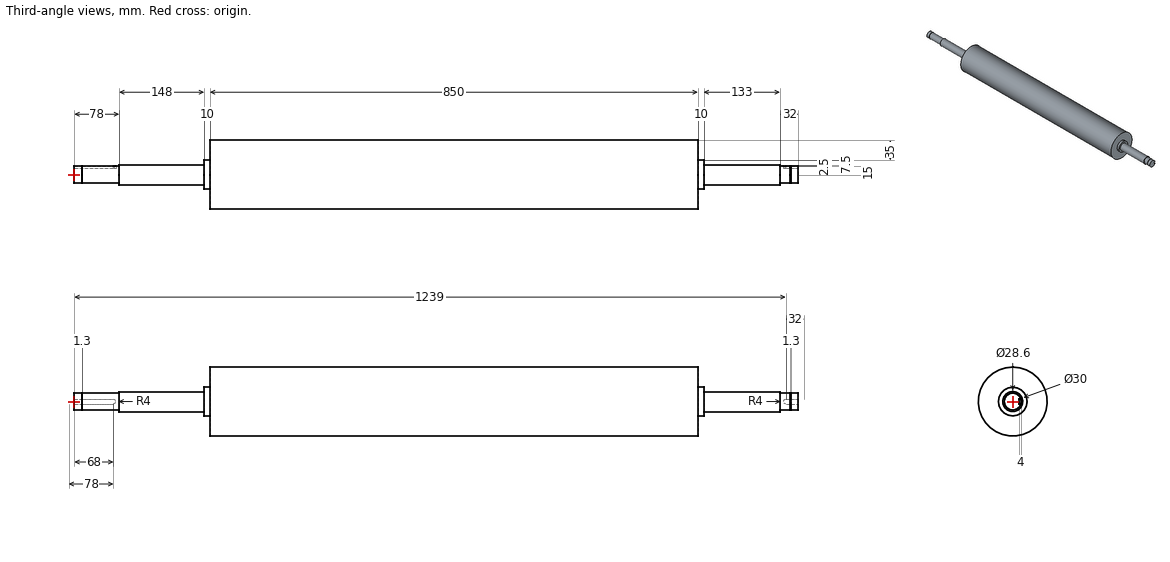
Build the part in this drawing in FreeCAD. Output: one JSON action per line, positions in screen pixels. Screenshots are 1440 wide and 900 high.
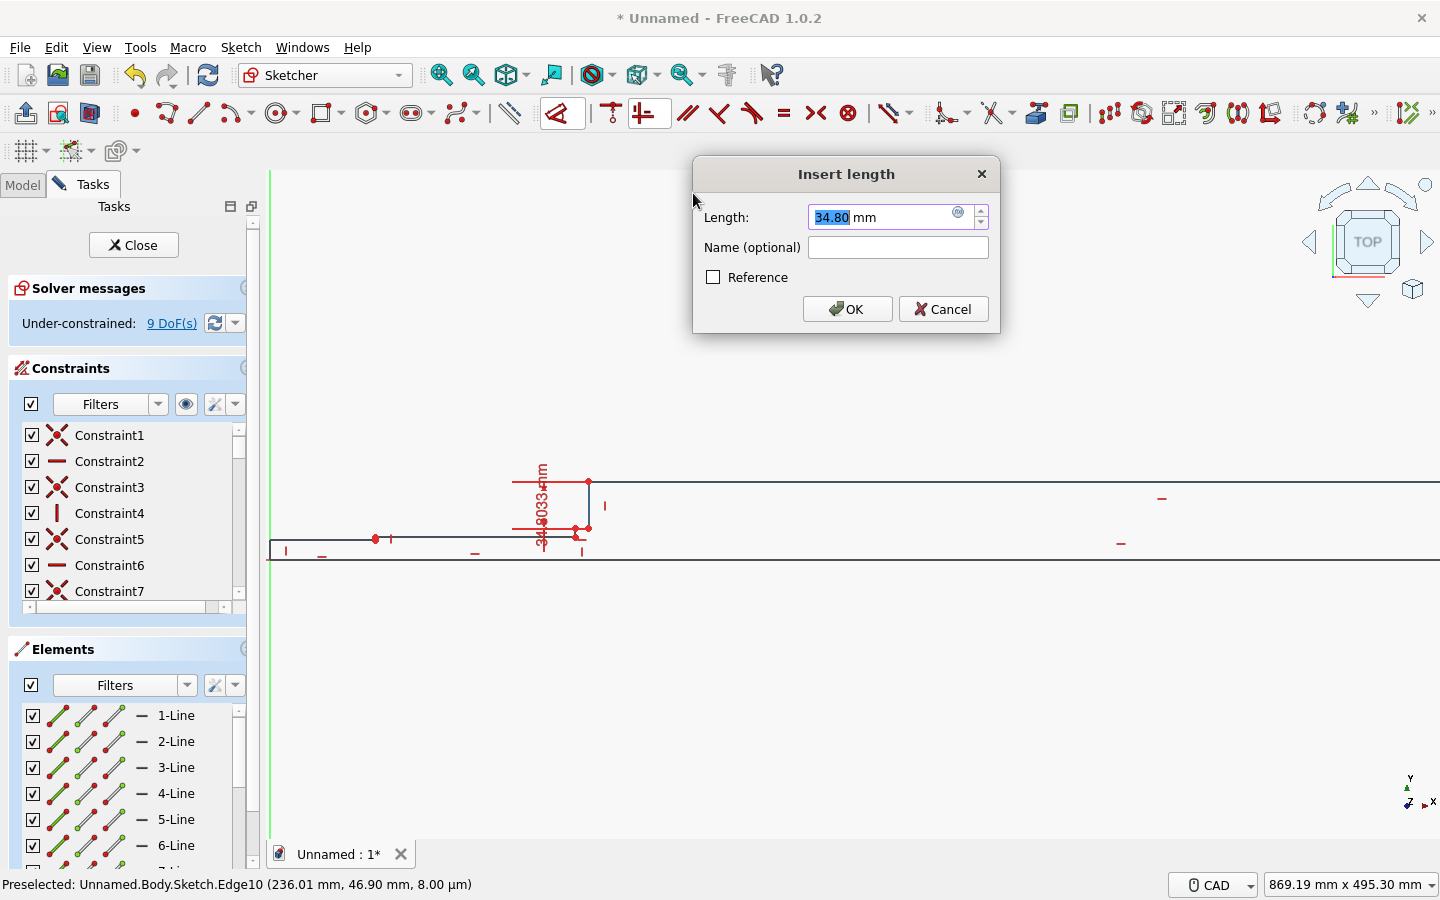
{"action": "type", "text": "35"}
{"action": "key", "text": "Return"}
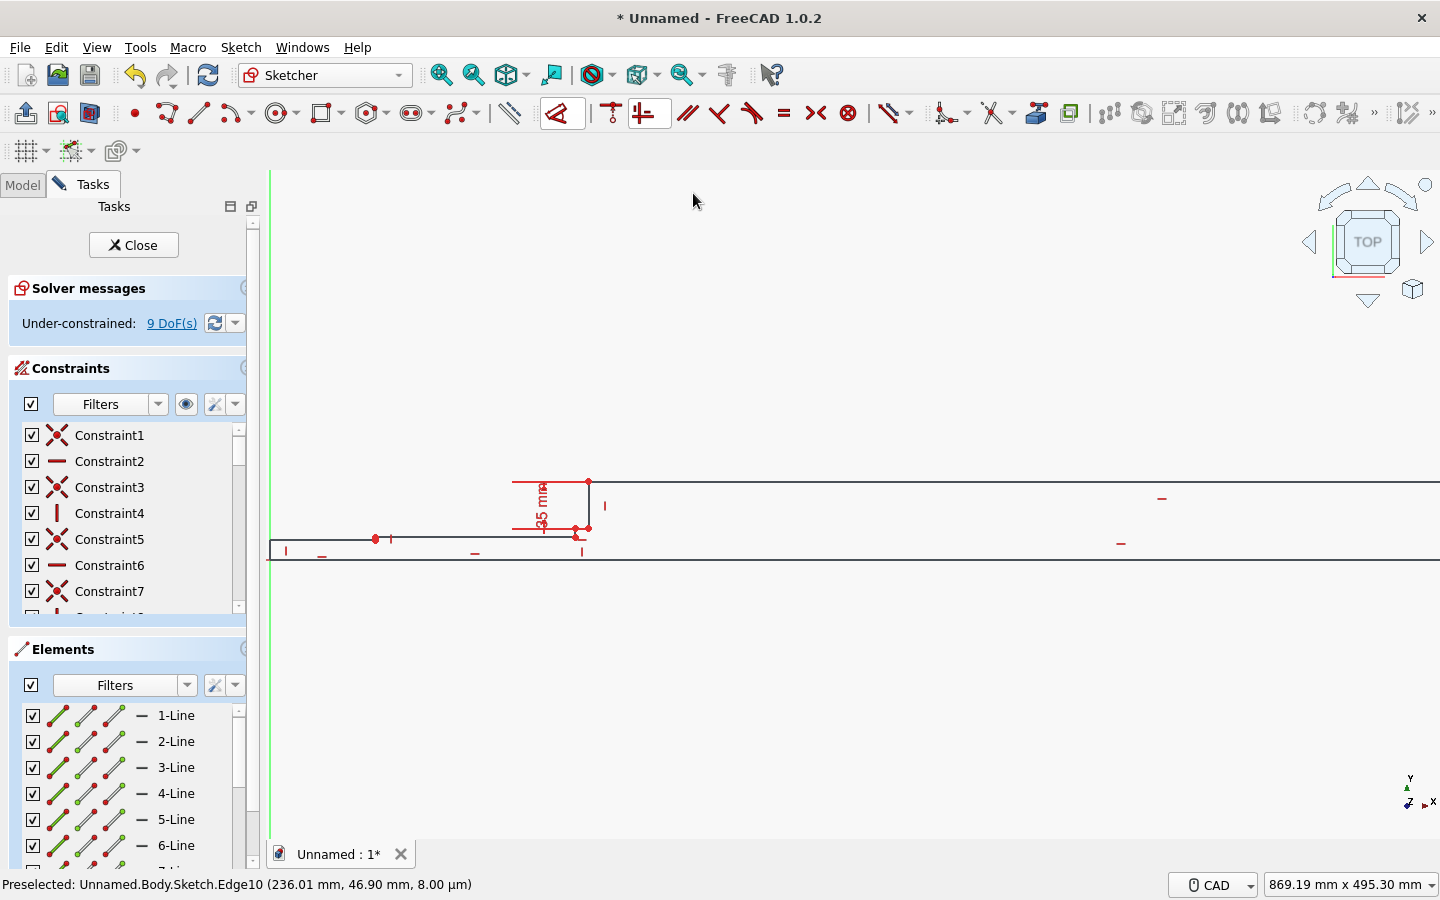
{"action": "scroll", "coordinate": [582, 529], "scroll_direction": "up", "scroll_amount": 6}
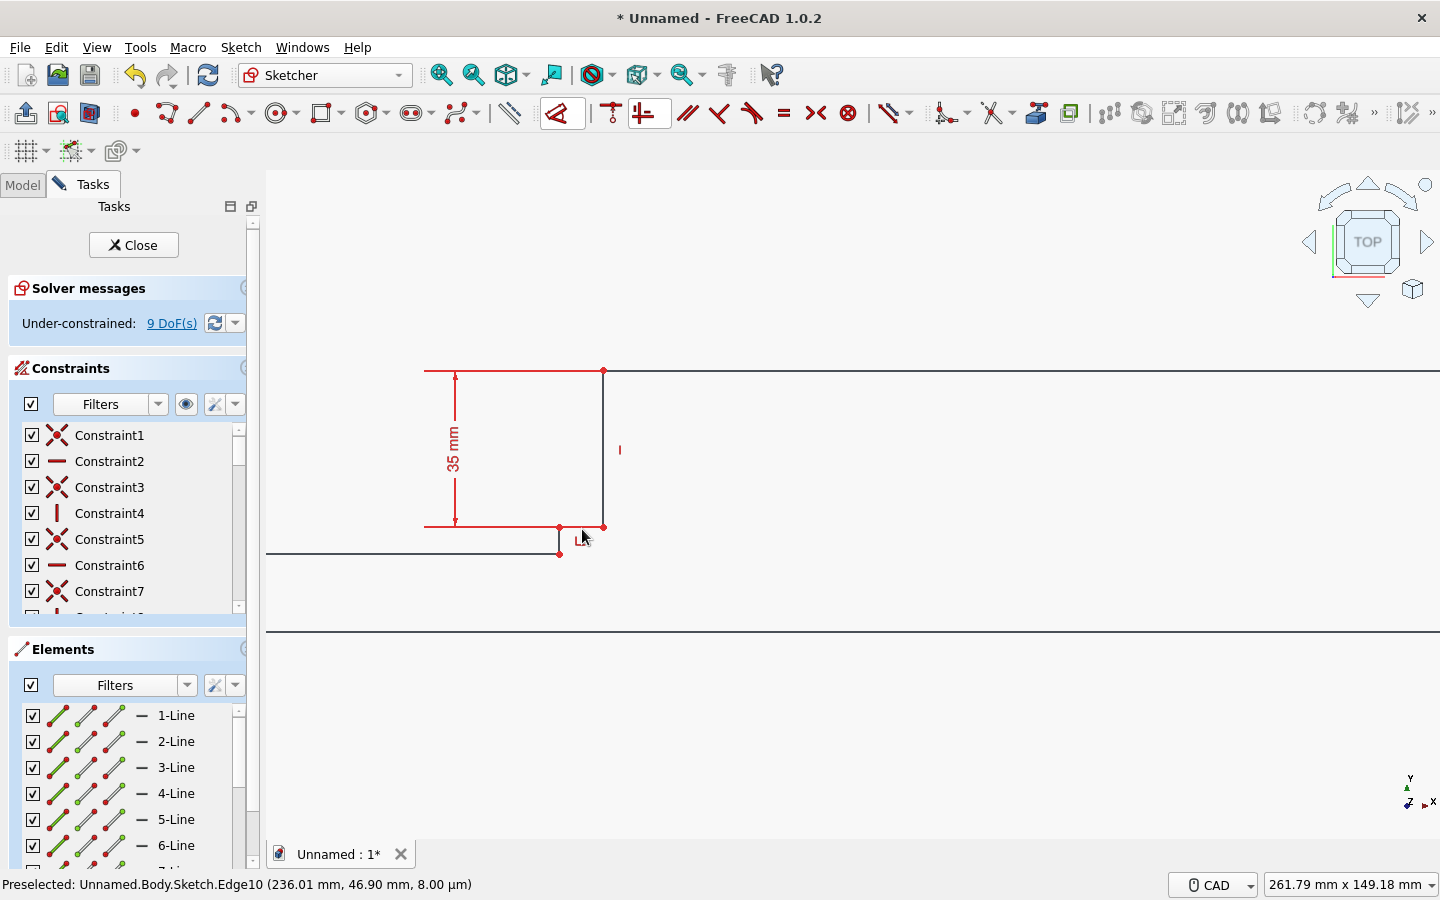
{"action": "left_click", "coordinate": [581, 527]}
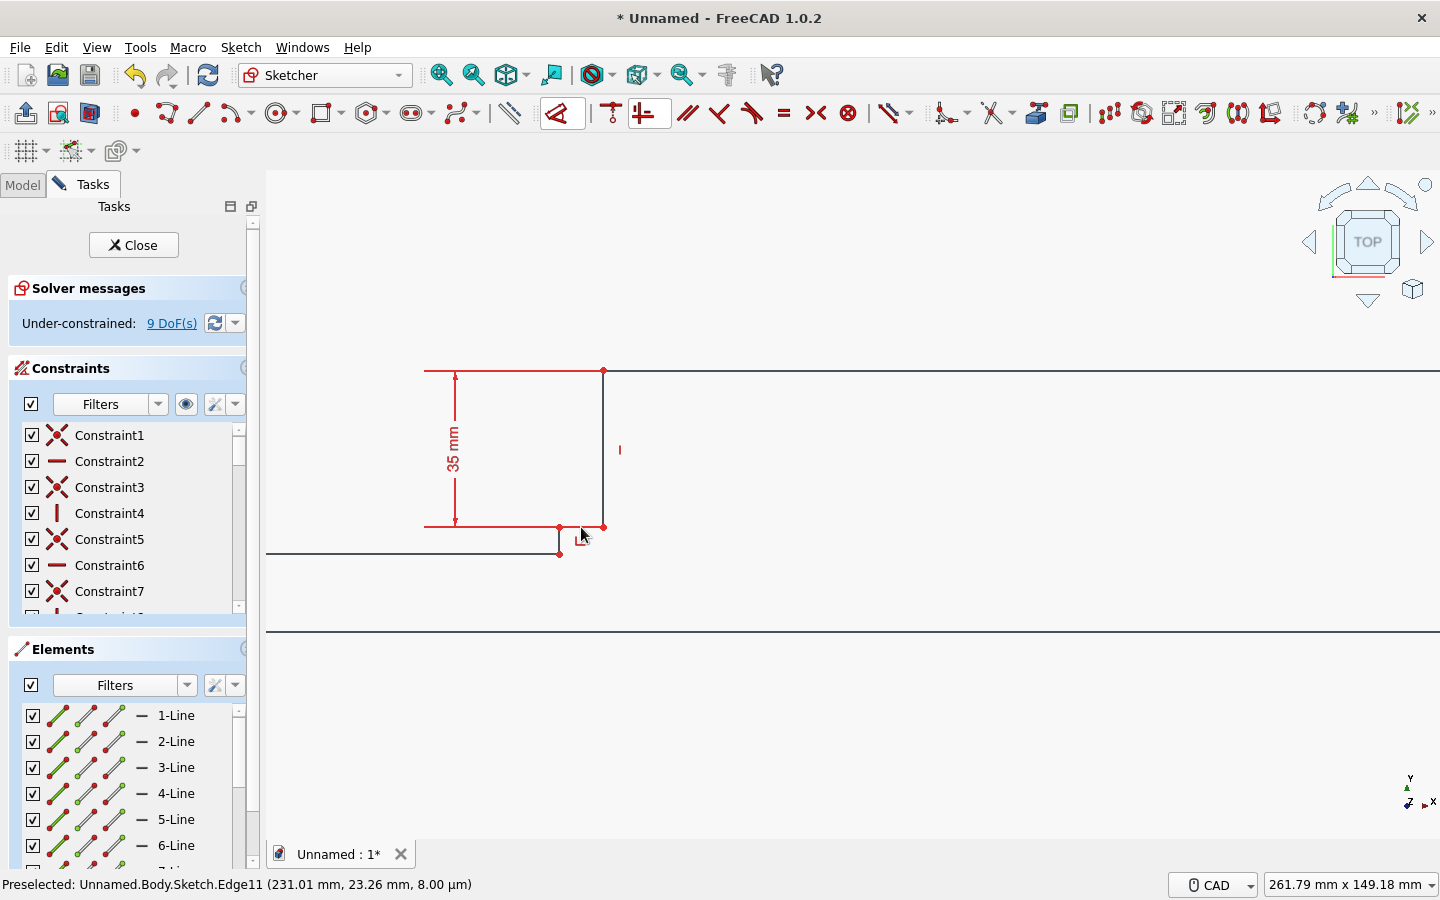
{"action": "key", "text": "l"}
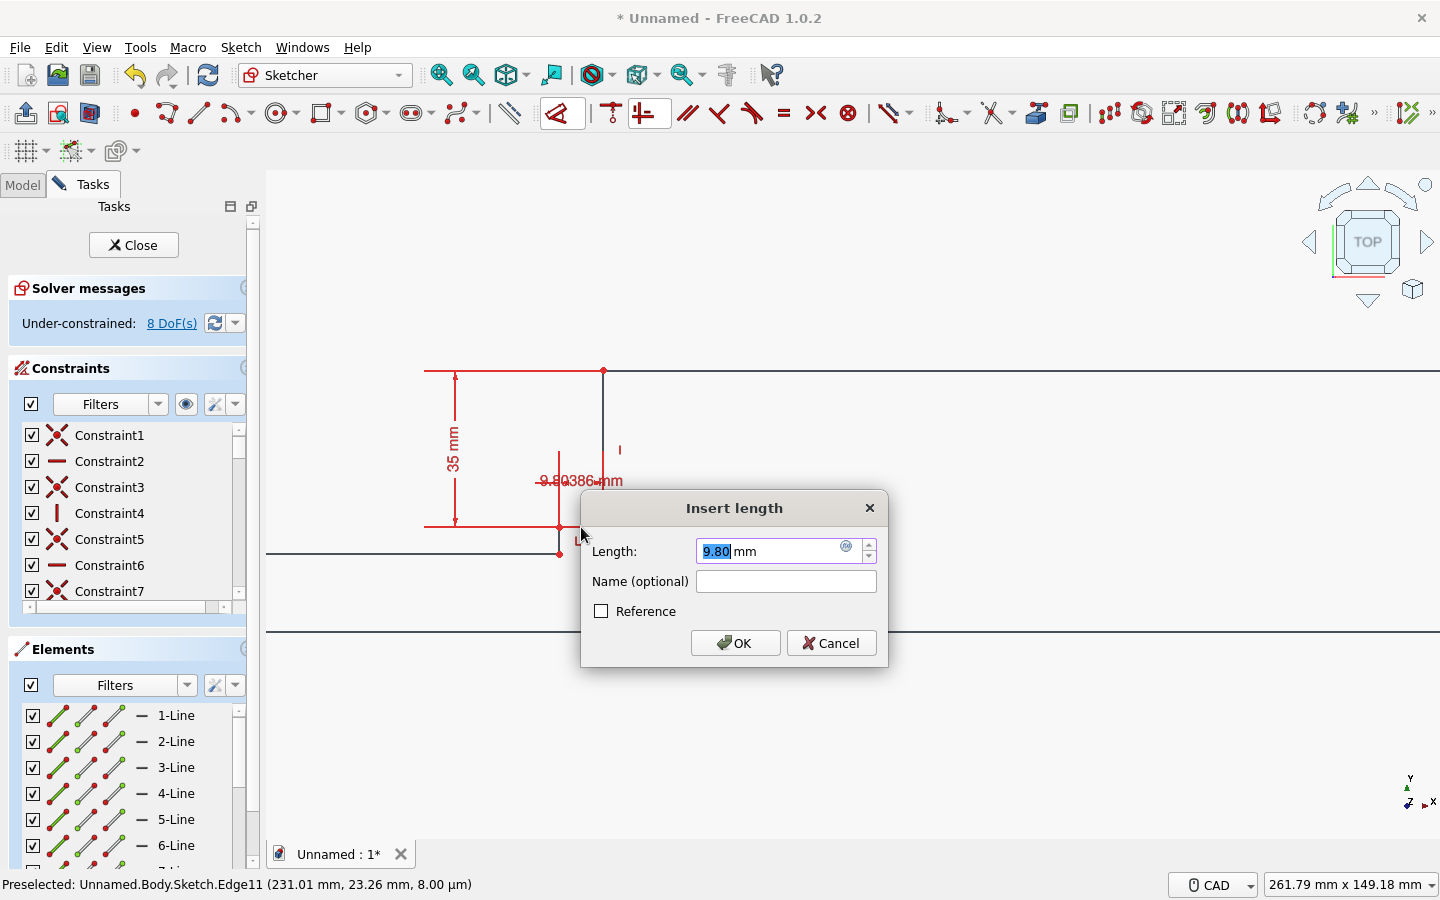
{"action": "type", "text": "10"}
{"action": "key", "text": "Return"}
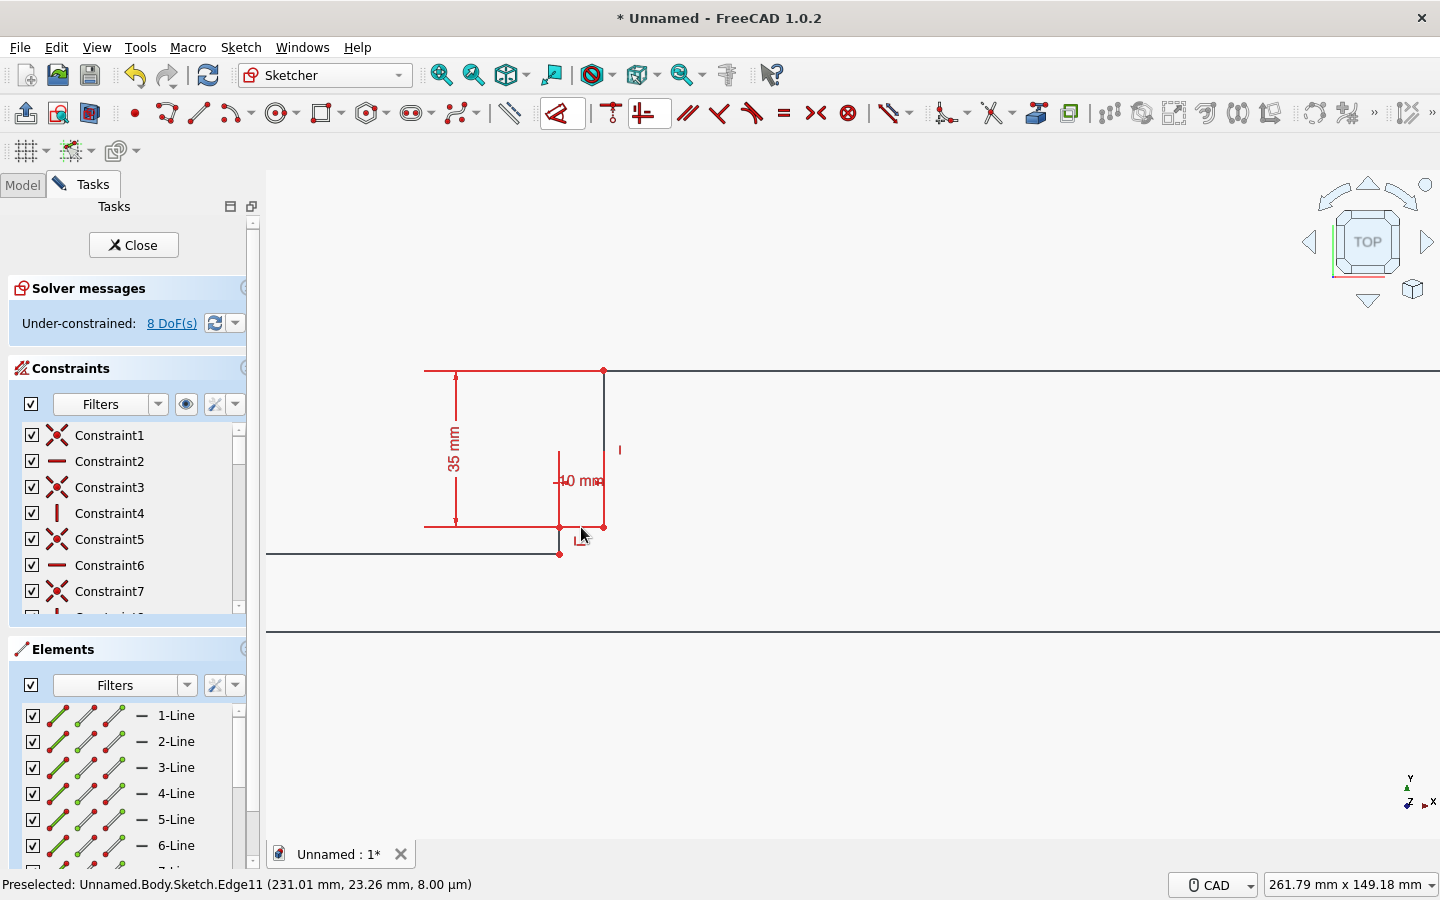
{"action": "scroll", "coordinate": [587, 505], "scroll_direction": "down", "scroll_amount": 11}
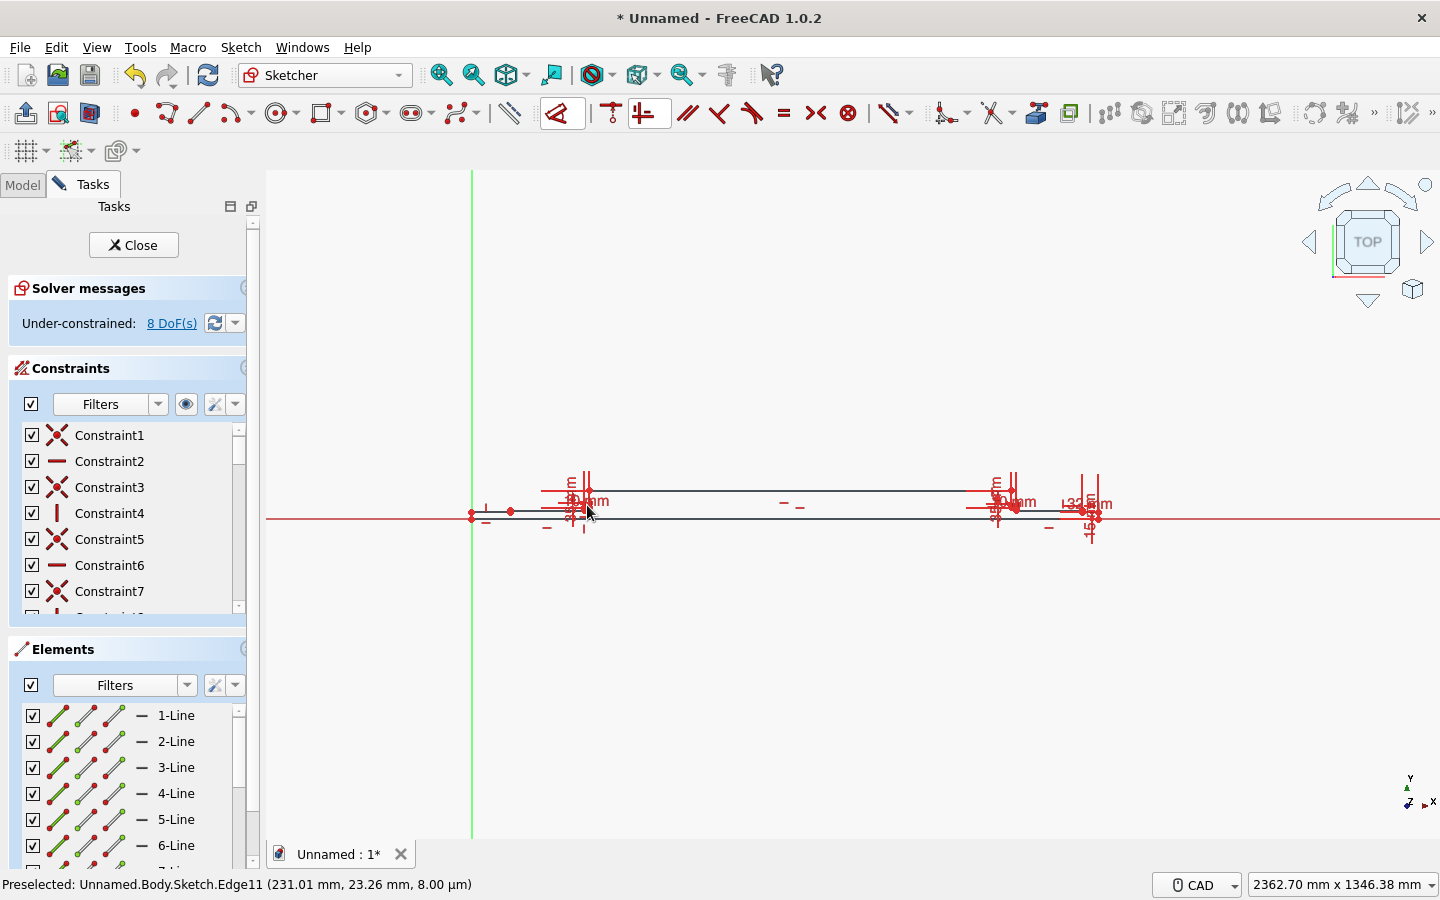
{"action": "scroll", "coordinate": [499, 512], "scroll_direction": "up", "scroll_amount": 4}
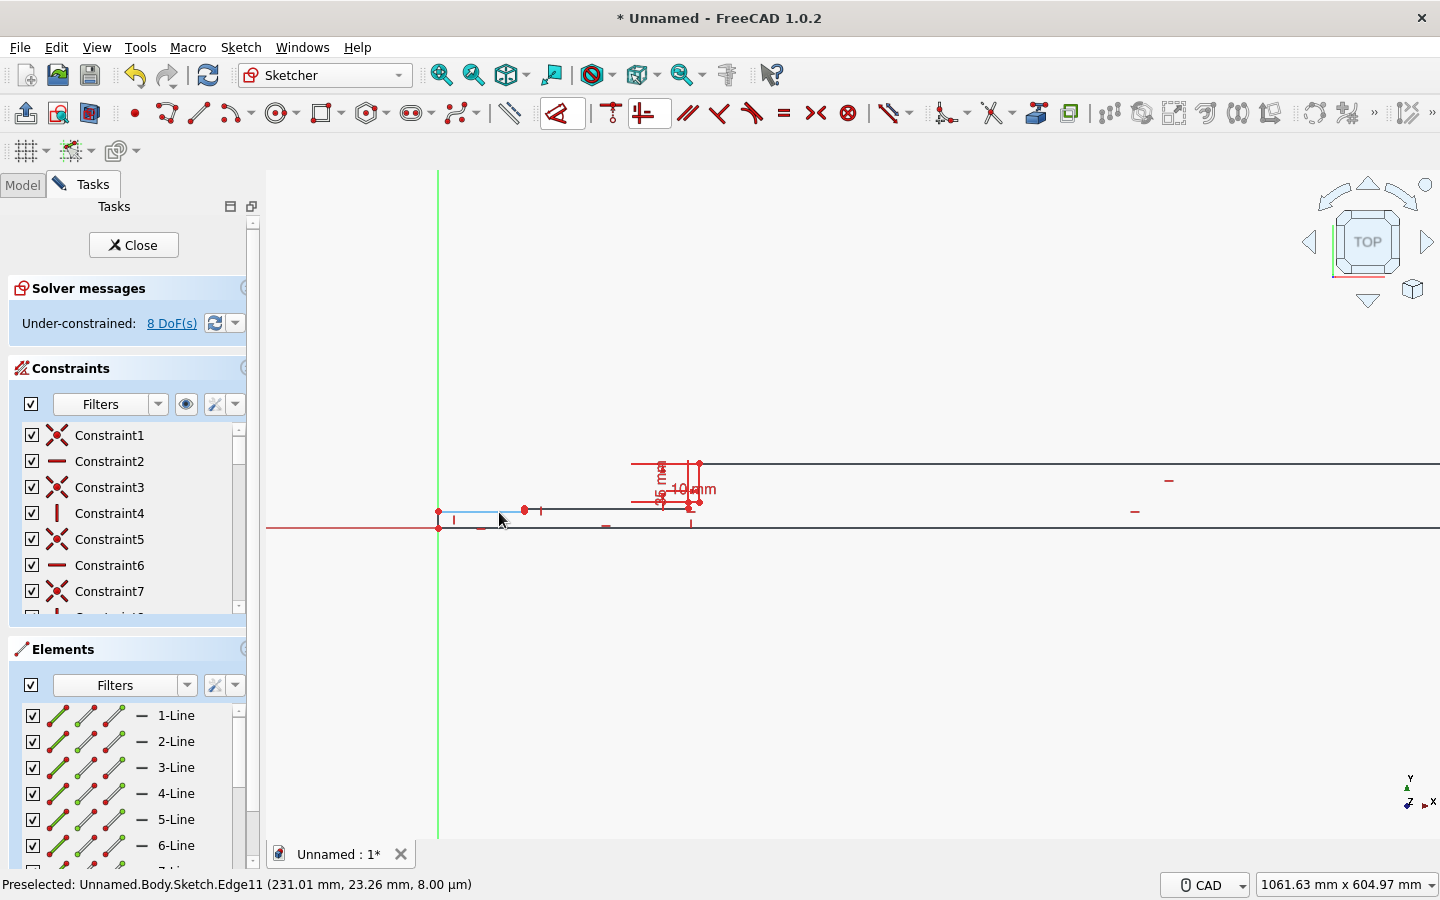
{"action": "left_click", "coordinate": [499, 512]}